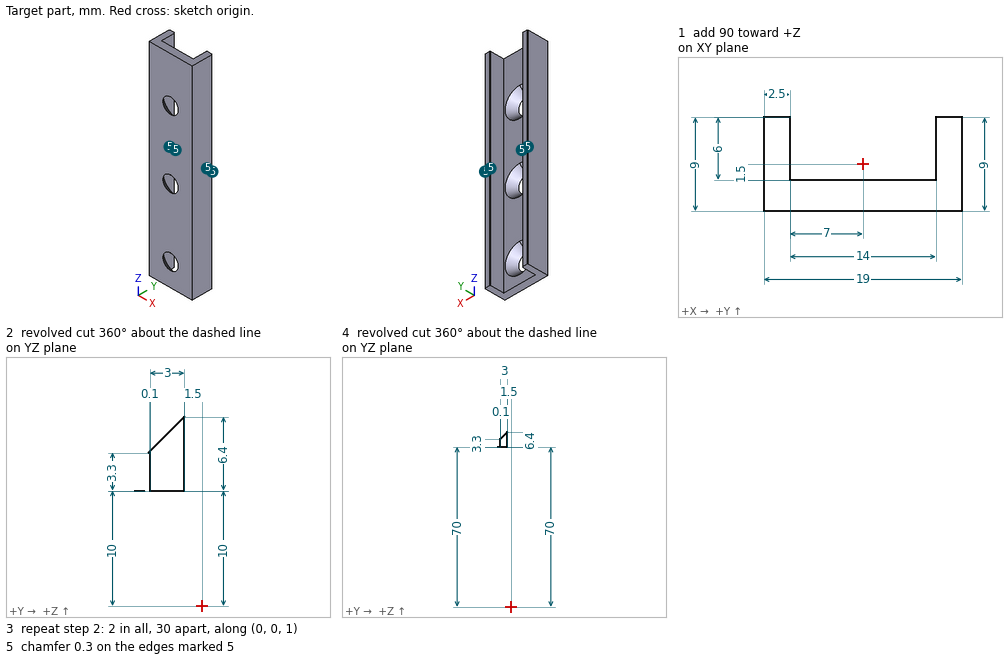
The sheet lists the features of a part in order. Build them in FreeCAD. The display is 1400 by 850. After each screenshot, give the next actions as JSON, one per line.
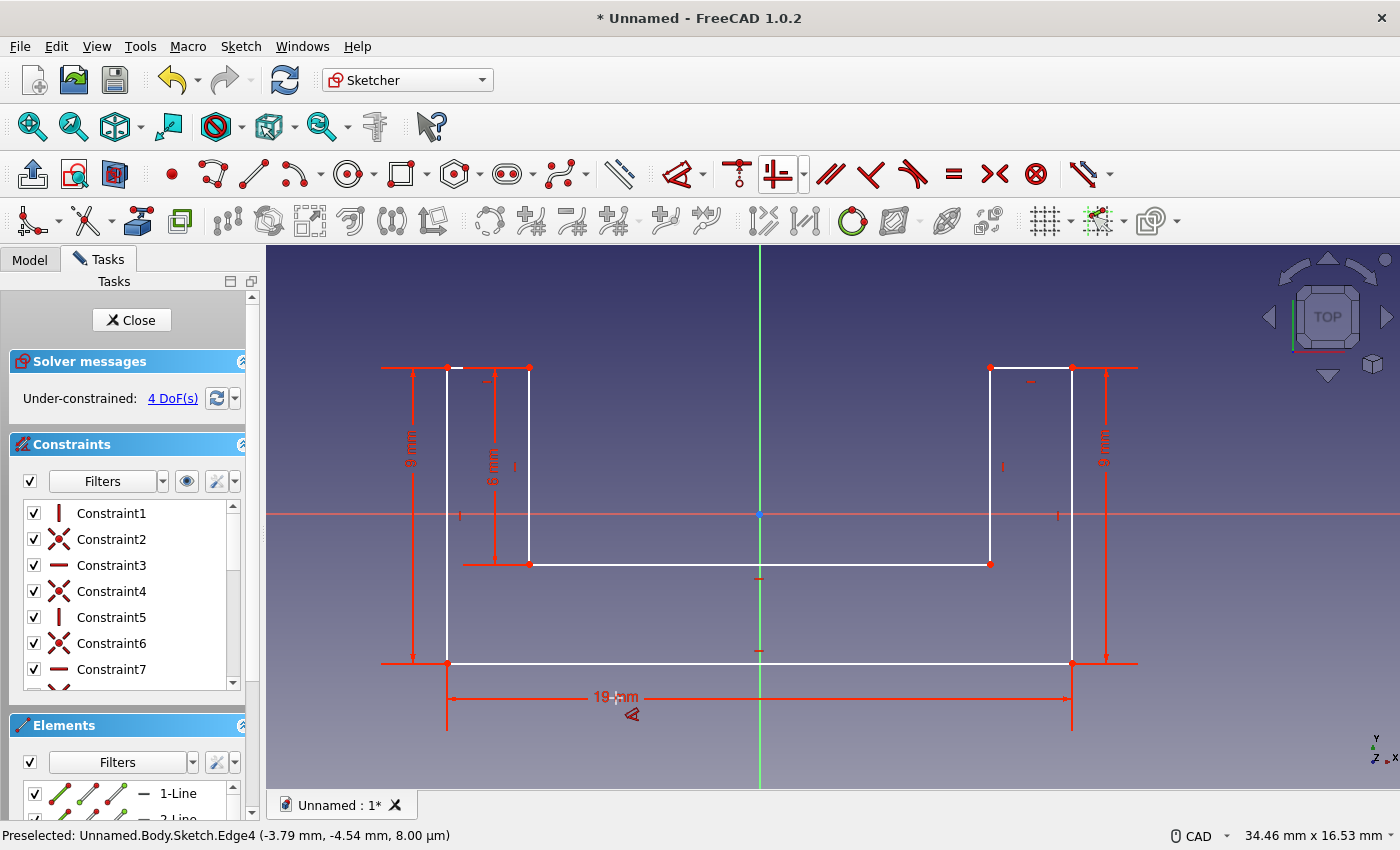
{"action": "left_click", "coordinate": [852, 565]}
{"action": "left_click", "coordinate": [653, 599]}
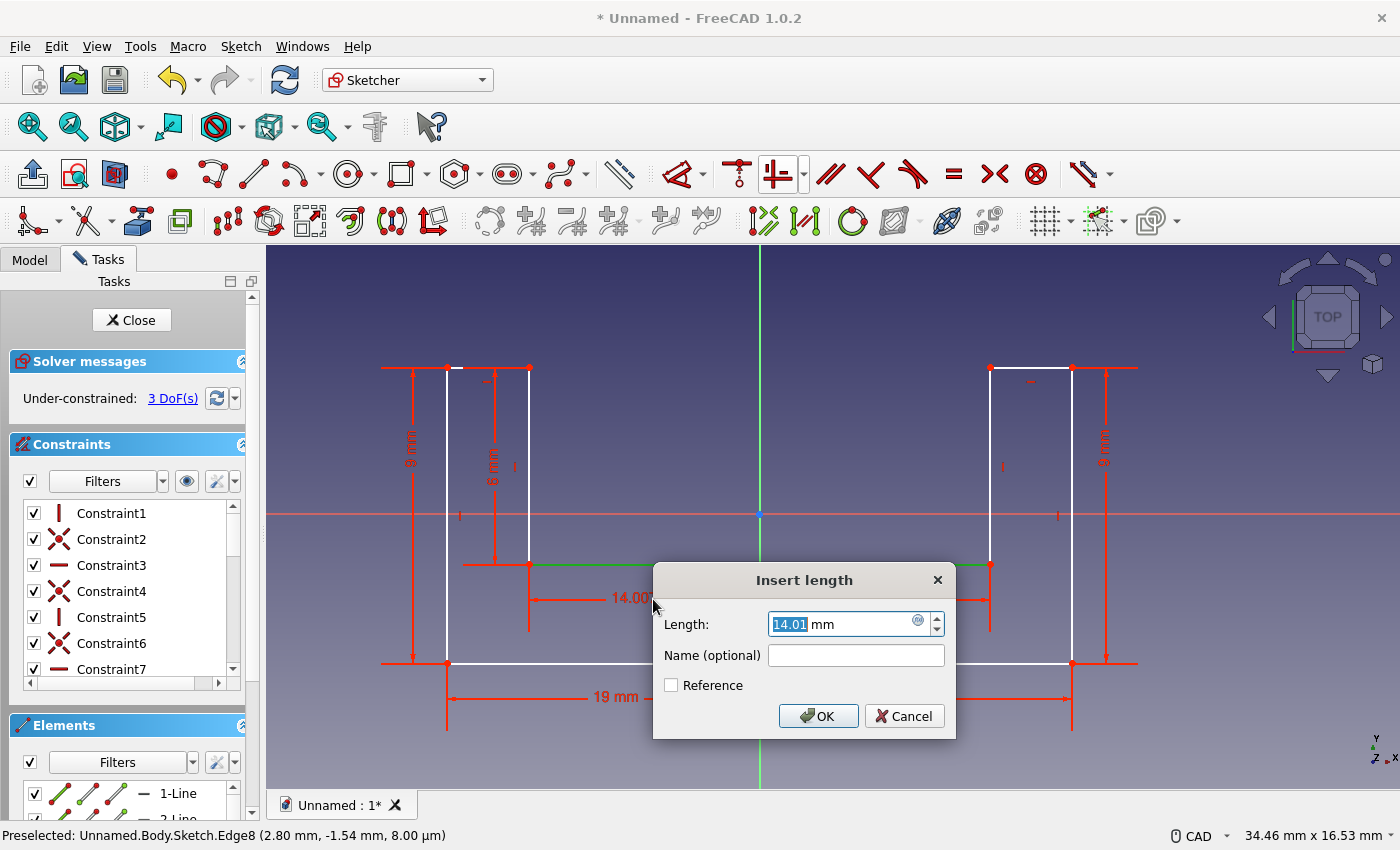
{"action": "type", "text": "14"}
{"action": "key", "text": "Return"}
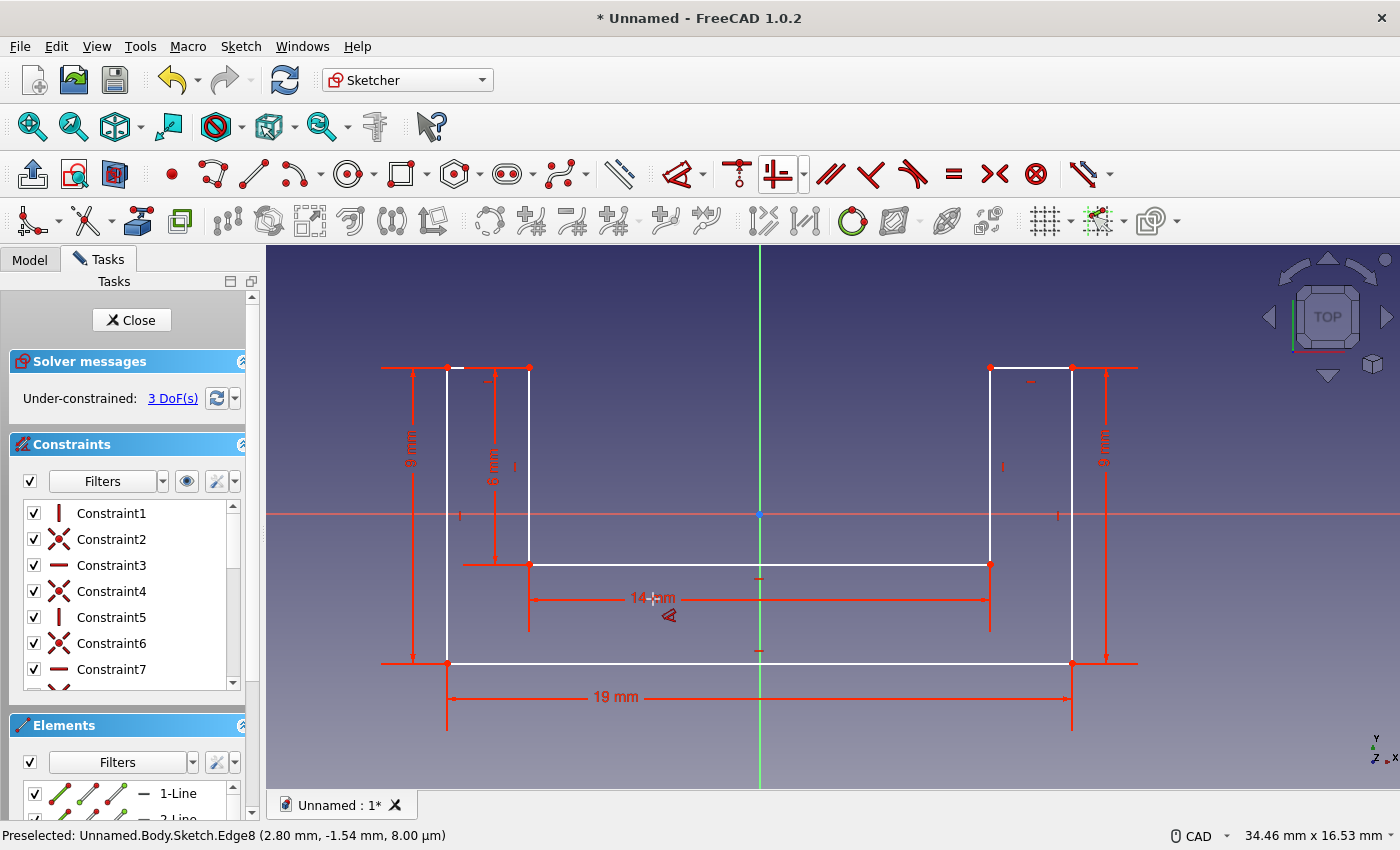
{"action": "left_click", "coordinate": [529, 565]}
{"action": "left_click", "coordinate": [564, 599]}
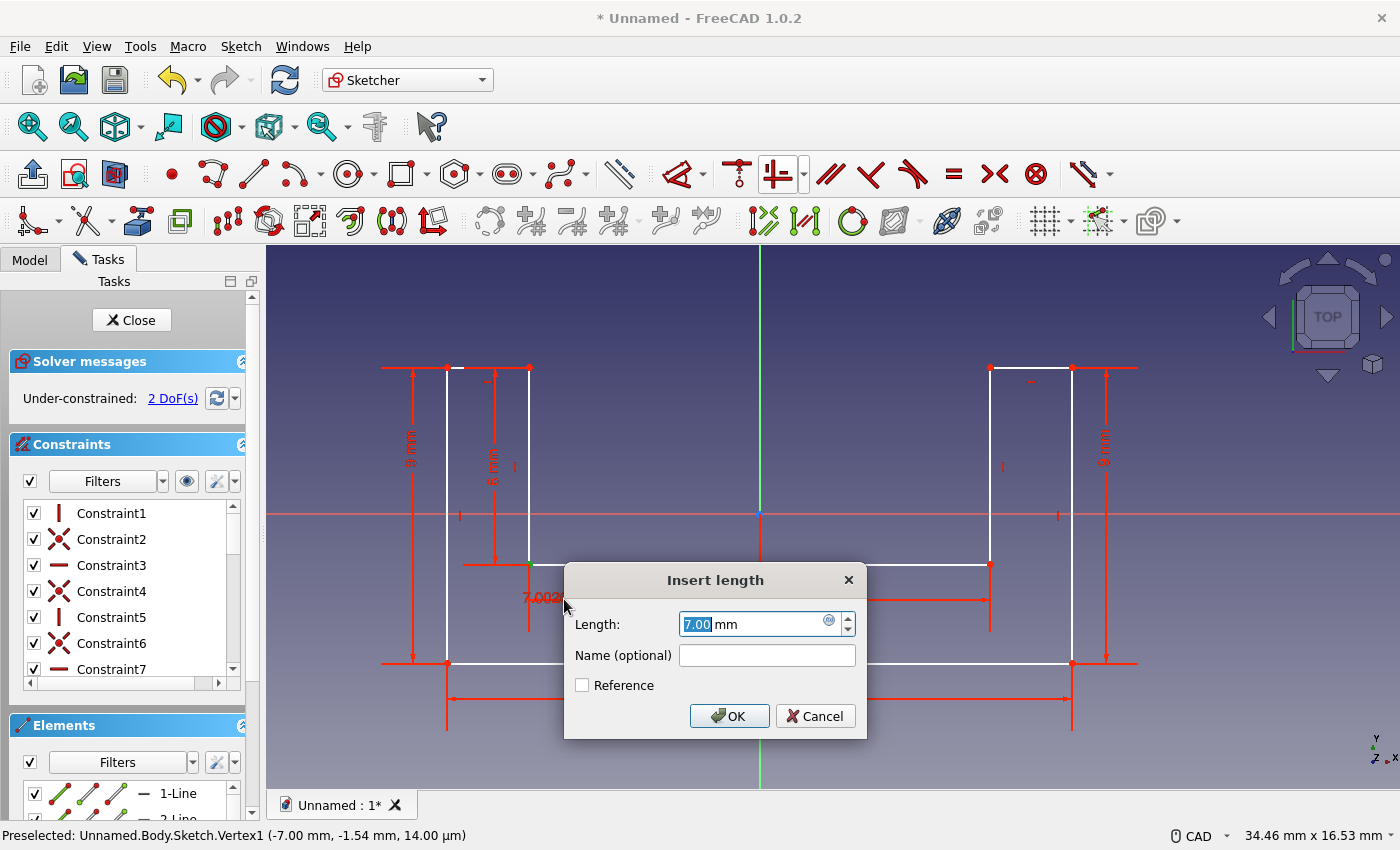
{"action": "type", "text": "7"}
{"action": "key", "text": "Return"}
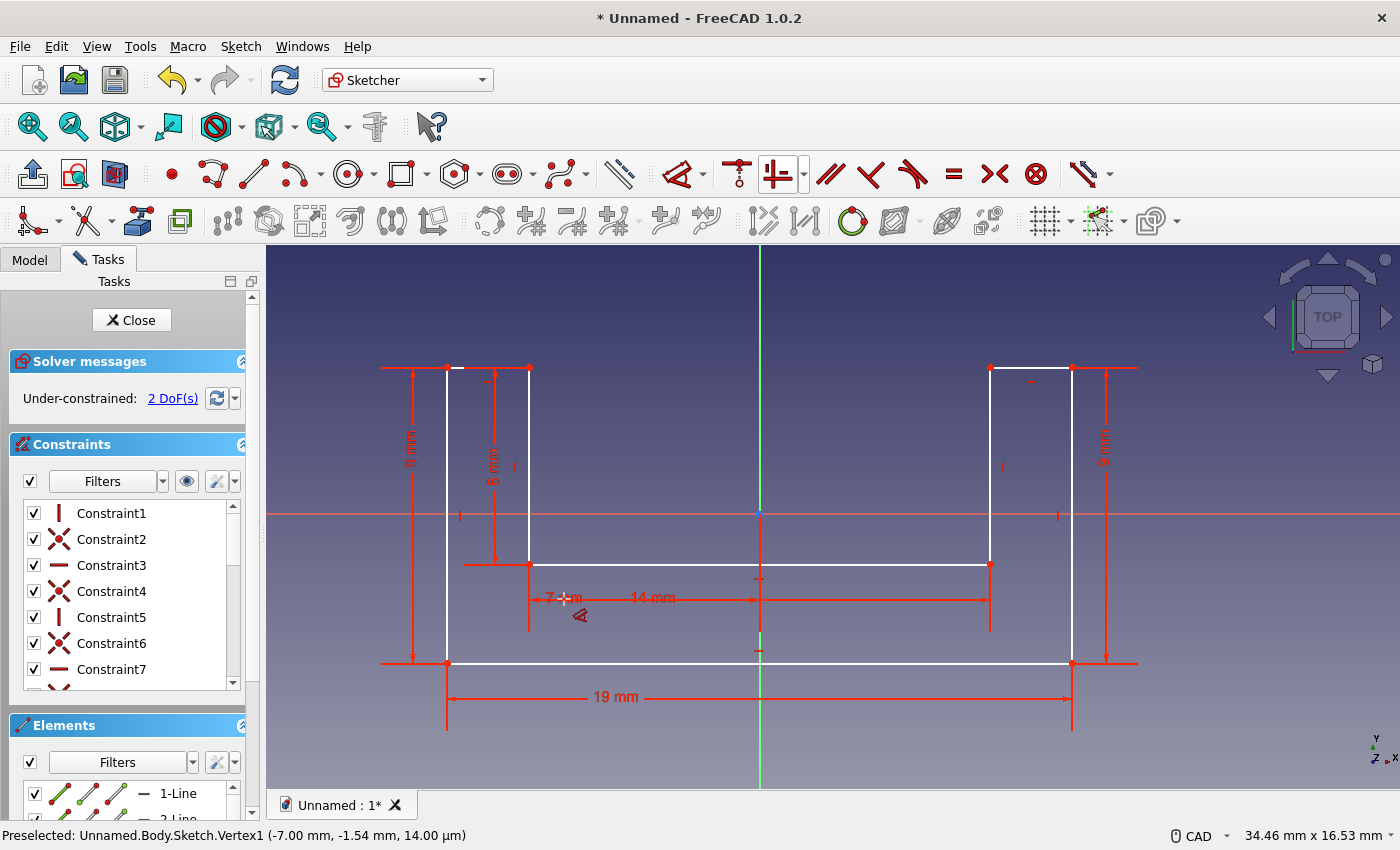
{"action": "left_click", "coordinate": [505, 368]}
{"action": "left_click", "coordinate": [488, 334]}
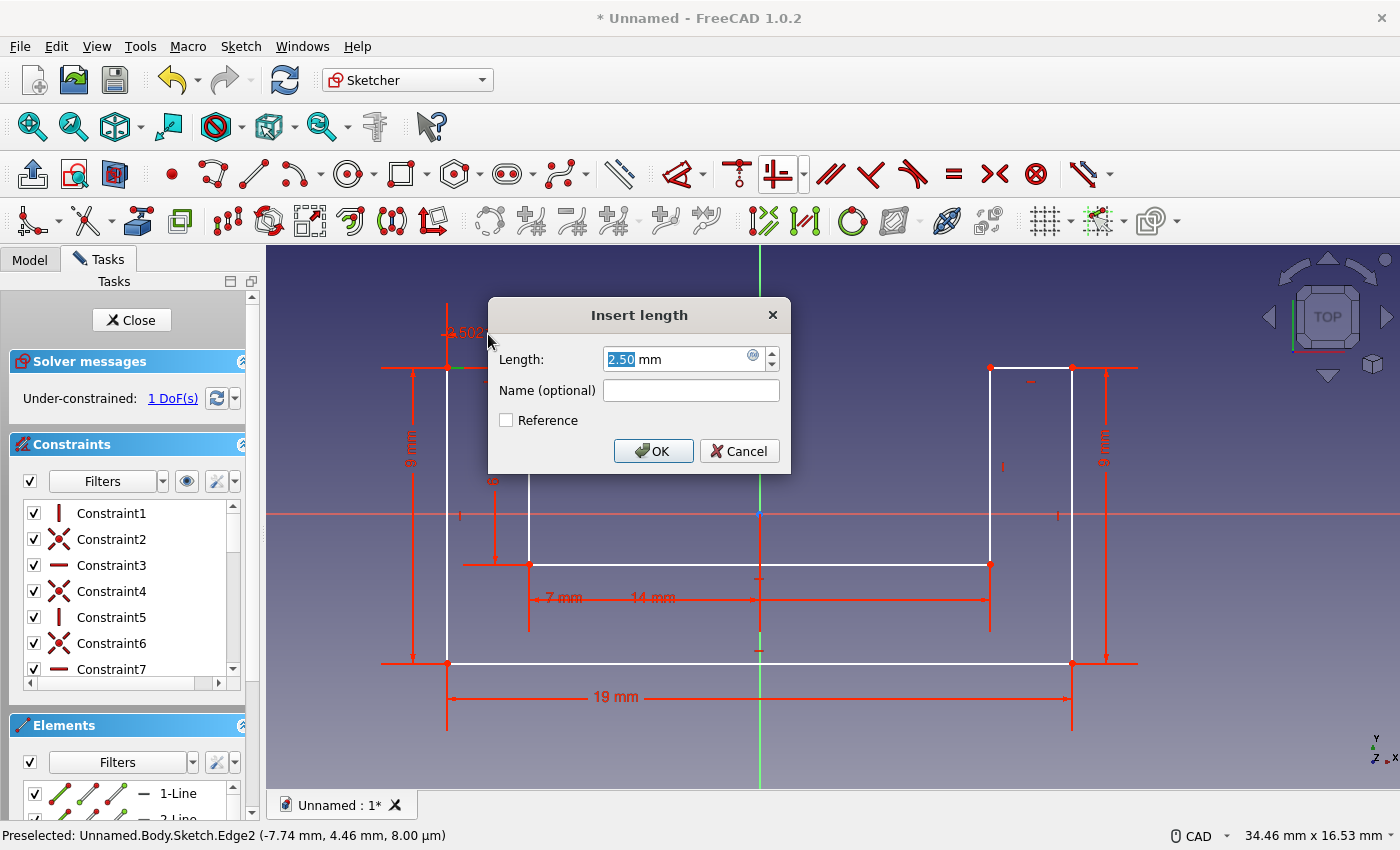
{"action": "type", "text": "2.5"}
{"action": "key", "text": "Return"}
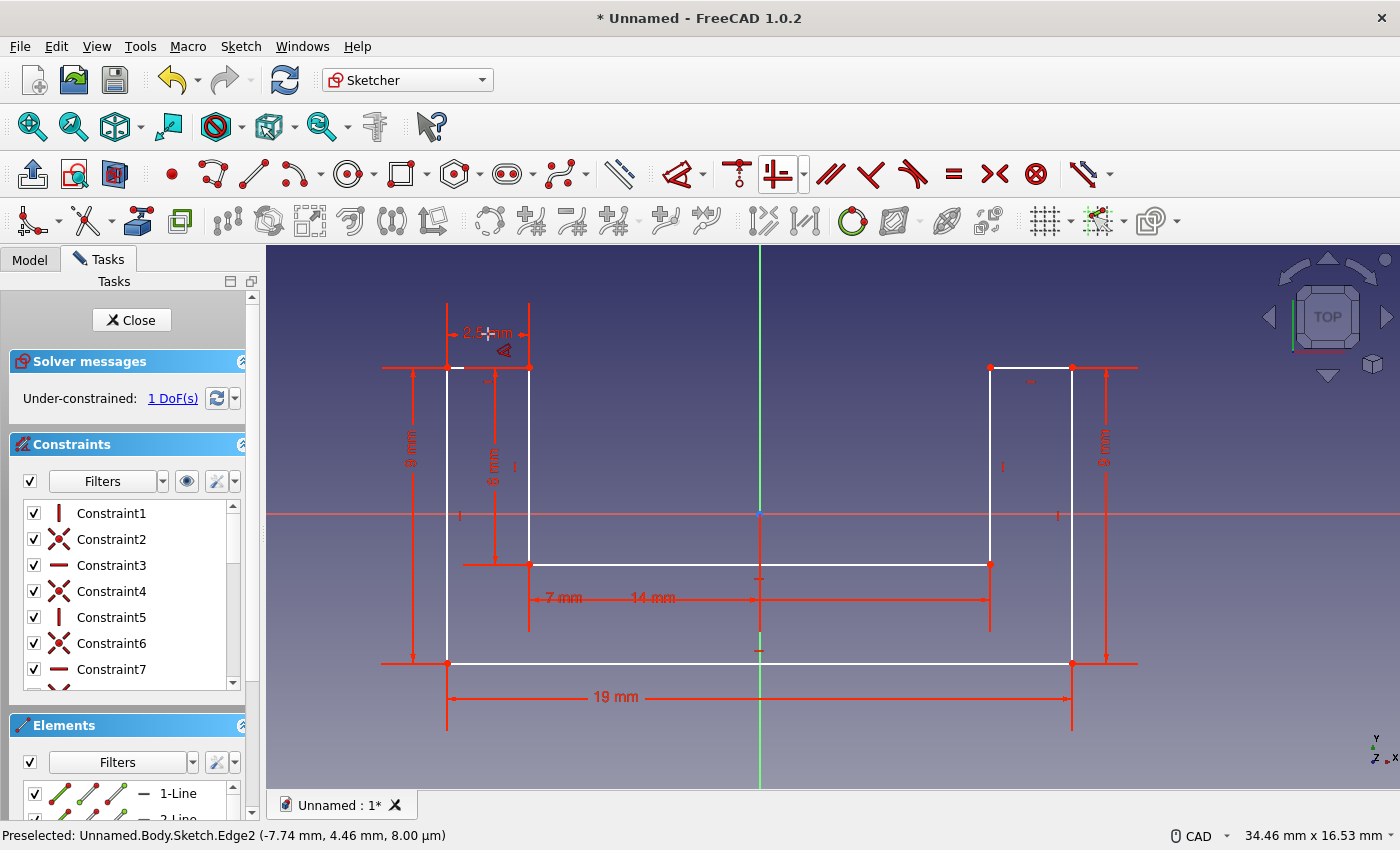
{"action": "left_click", "coordinate": [529, 565]}
{"action": "left_click", "coordinate": [495, 540]}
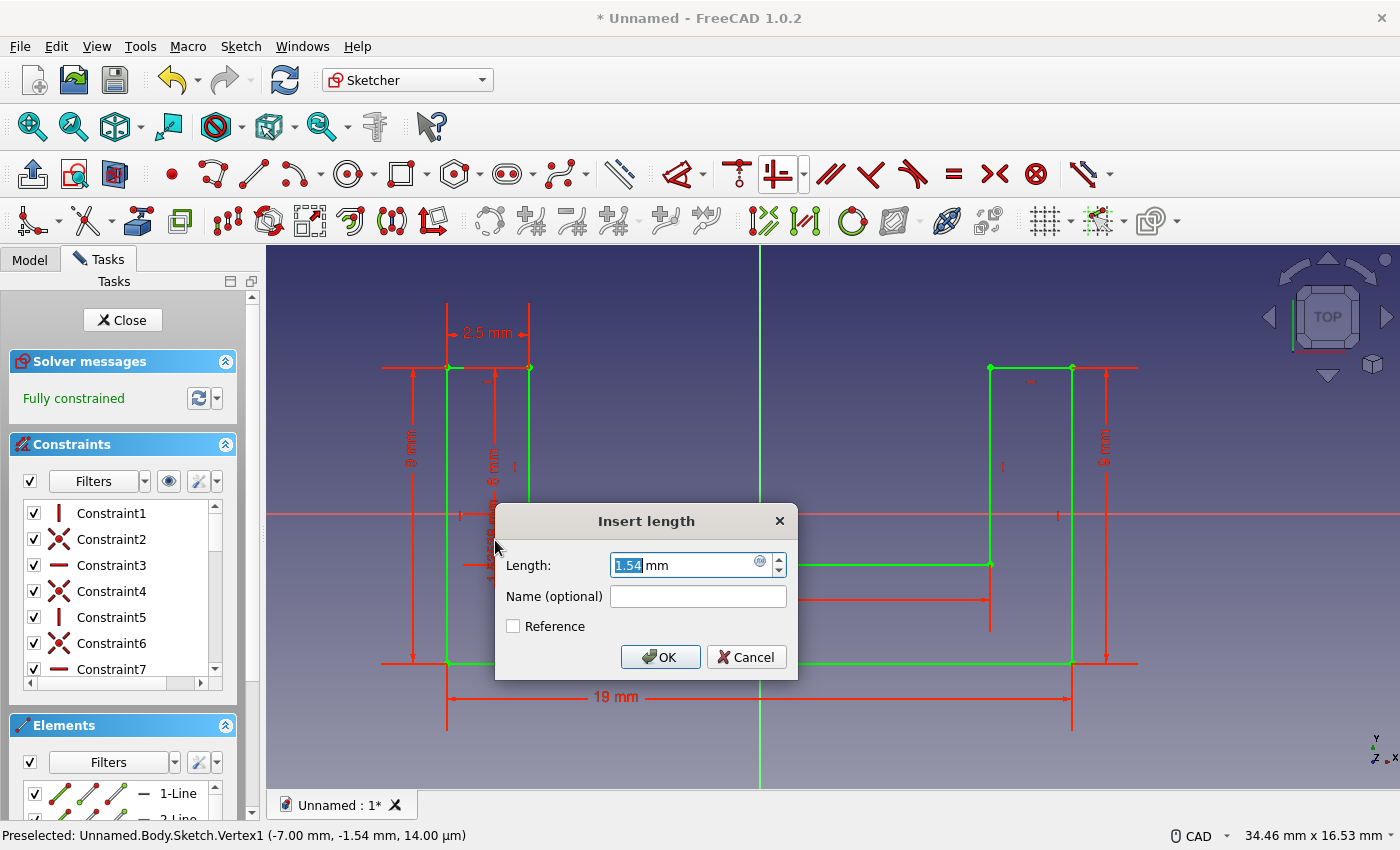
{"action": "type", "text": "1.5"}
{"action": "key", "text": "Return"}
{"action": "key", "text": "Escape"}